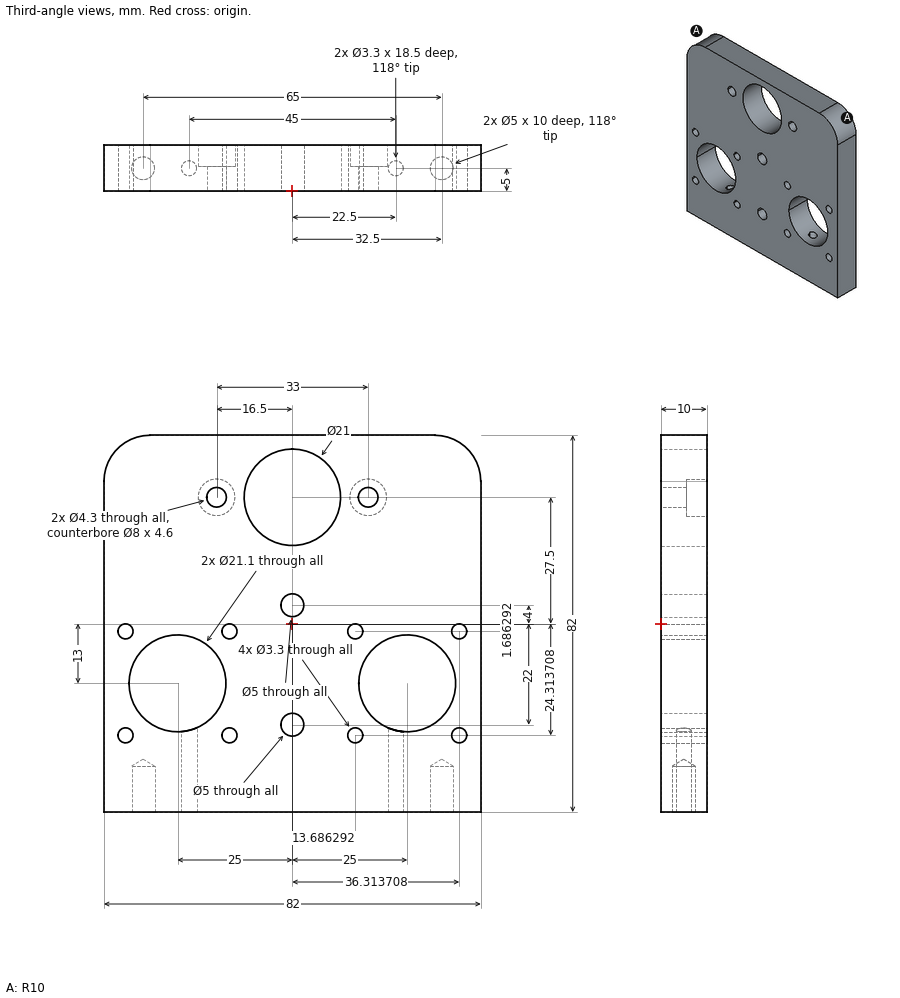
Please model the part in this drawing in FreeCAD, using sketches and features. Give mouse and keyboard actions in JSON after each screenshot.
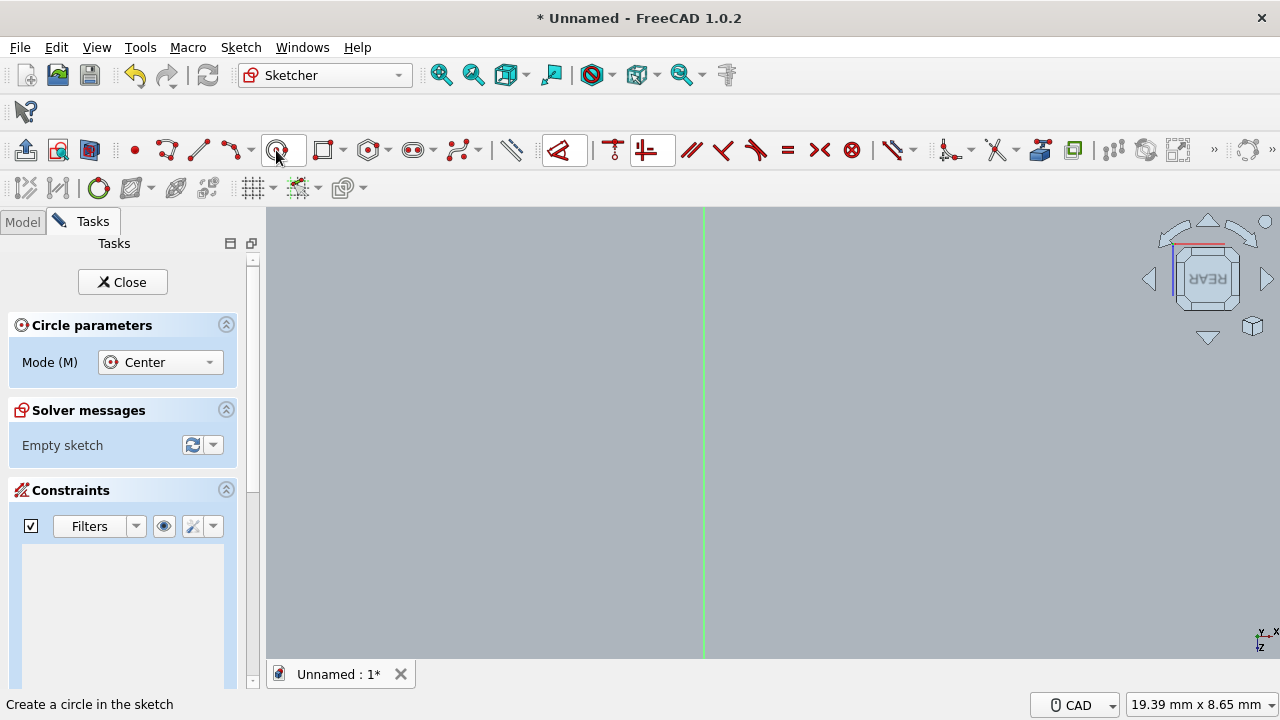
{"action": "left_click", "coordinate": [704, 426]}
{"action": "left_click", "coordinate": [797, 333]}
{"action": "key", "text": "Escape"}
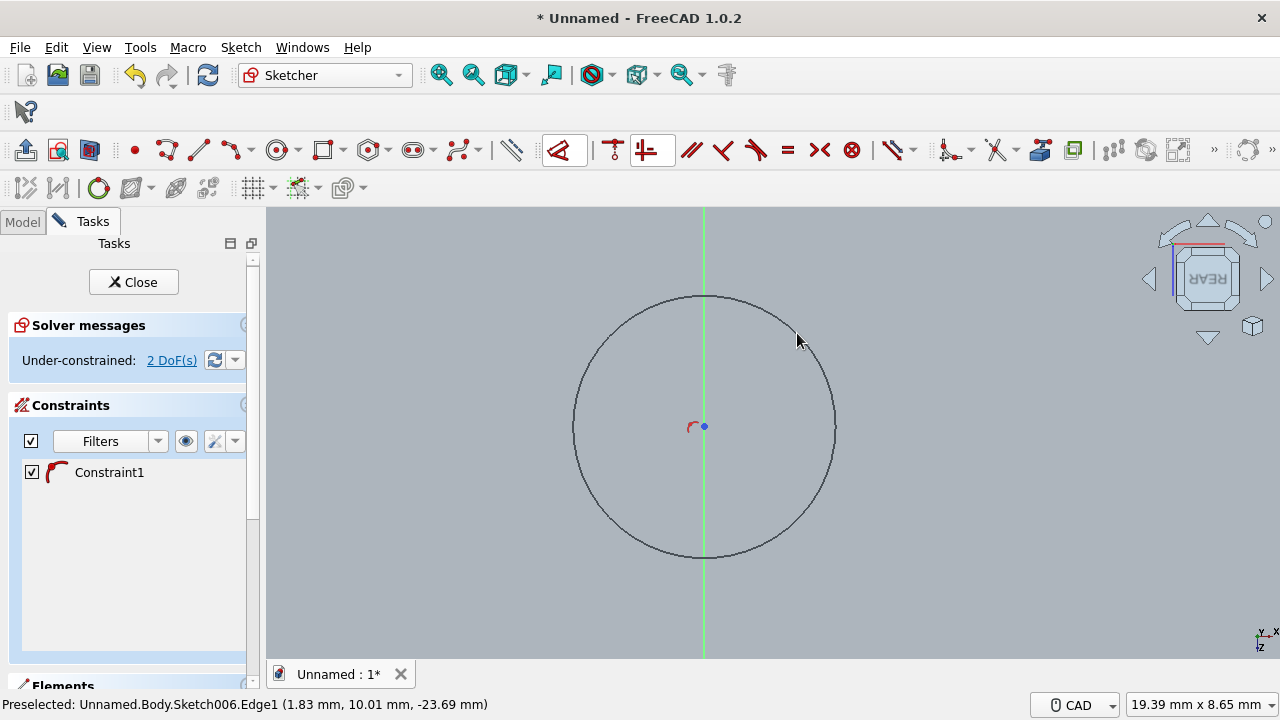
{"action": "left_click", "coordinate": [797, 334]}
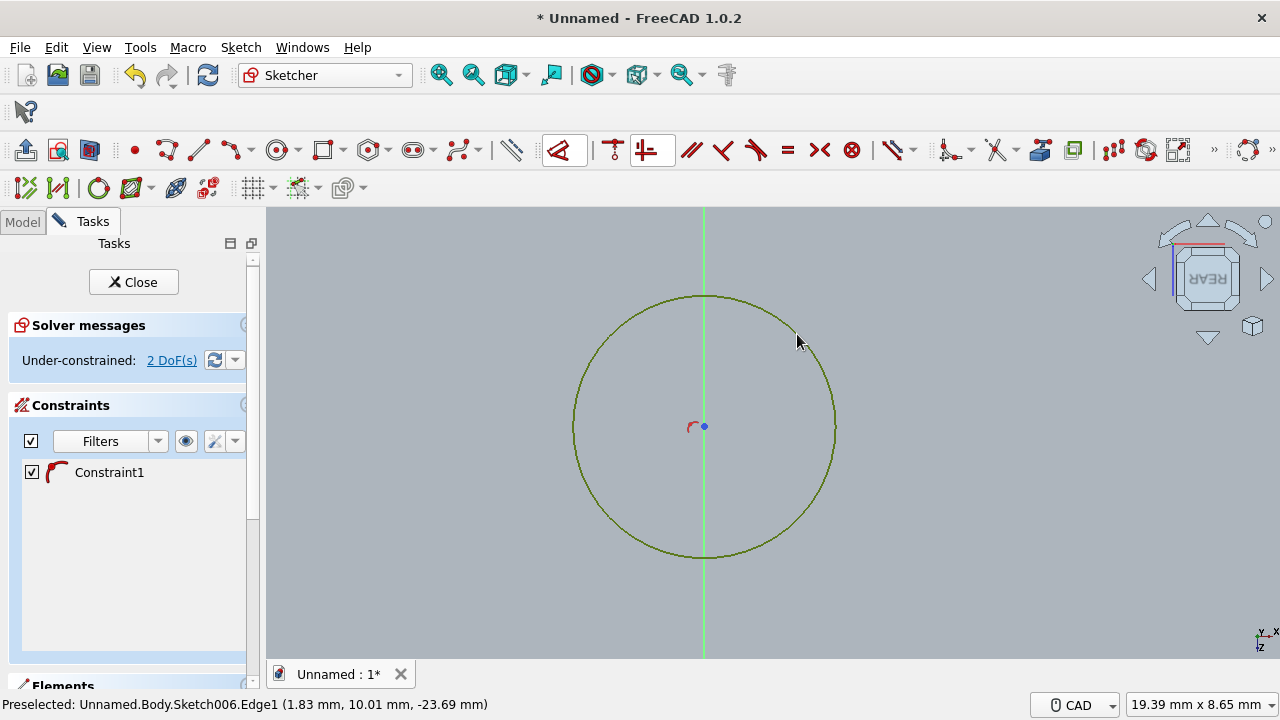
{"action": "left_click", "coordinate": [582, 150]}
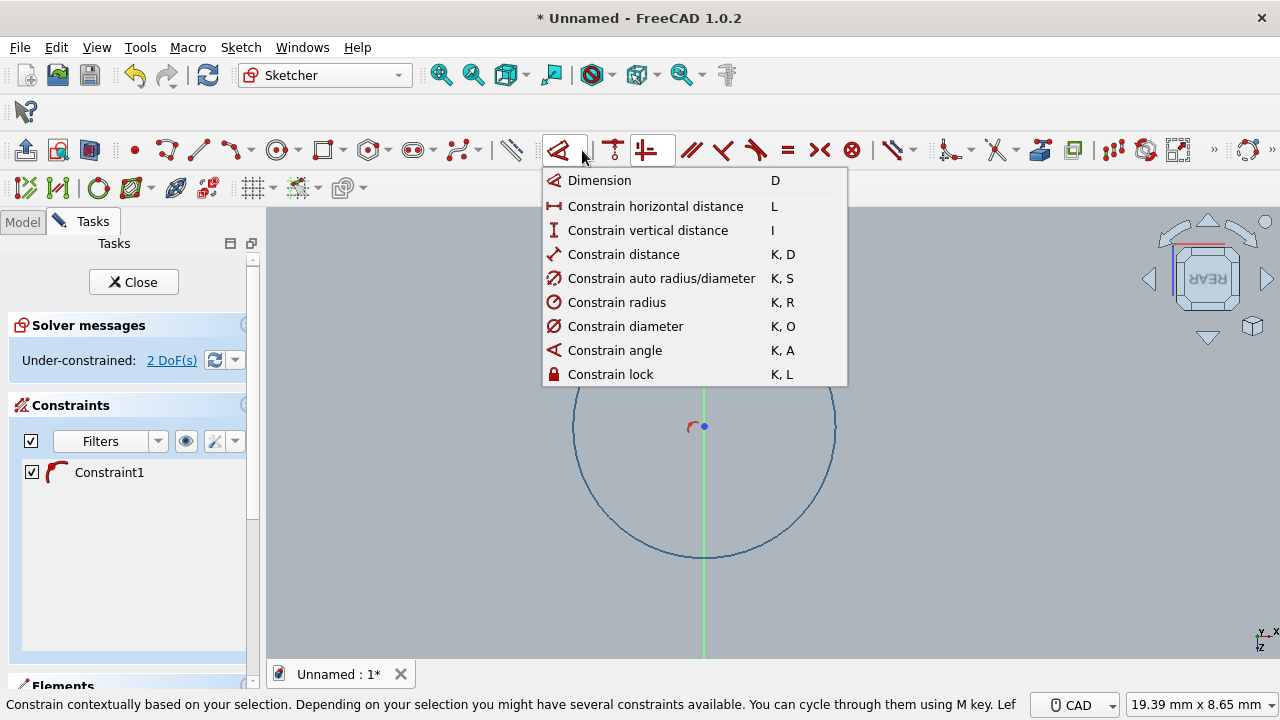
{"action": "left_click", "coordinate": [695, 326]}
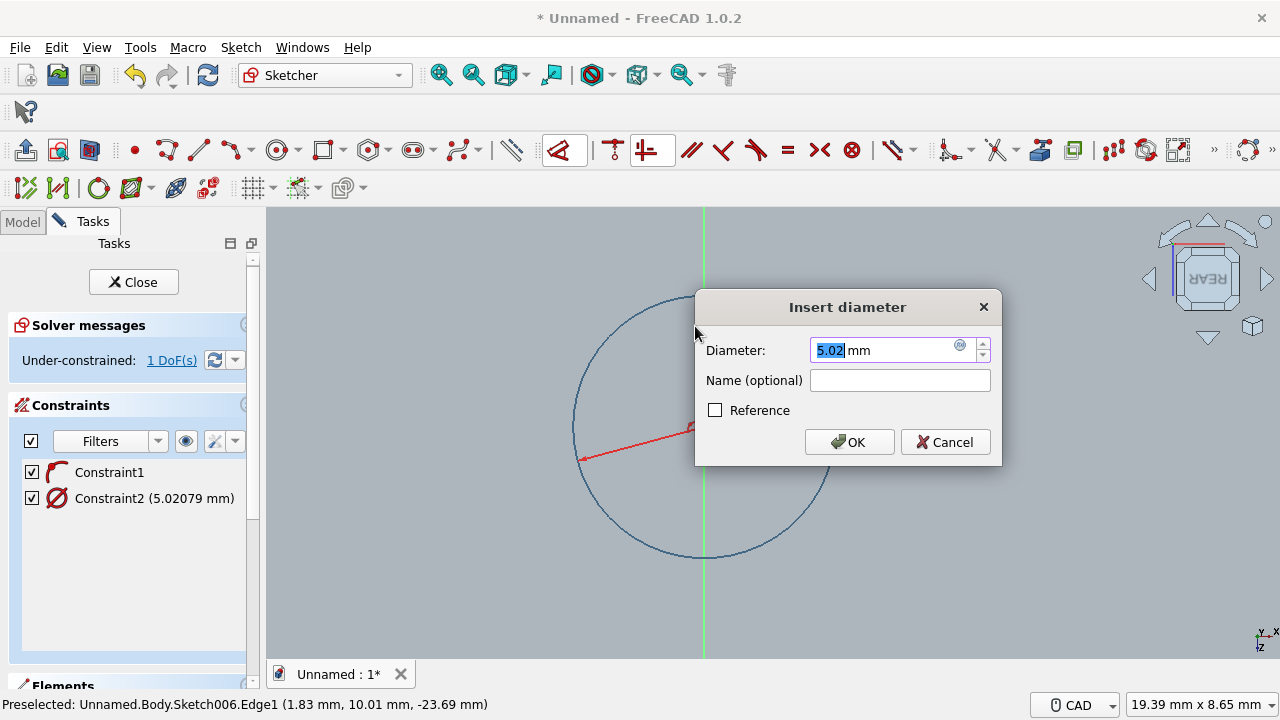
{"action": "type", "text": "5"}
{"action": "key", "text": "Return"}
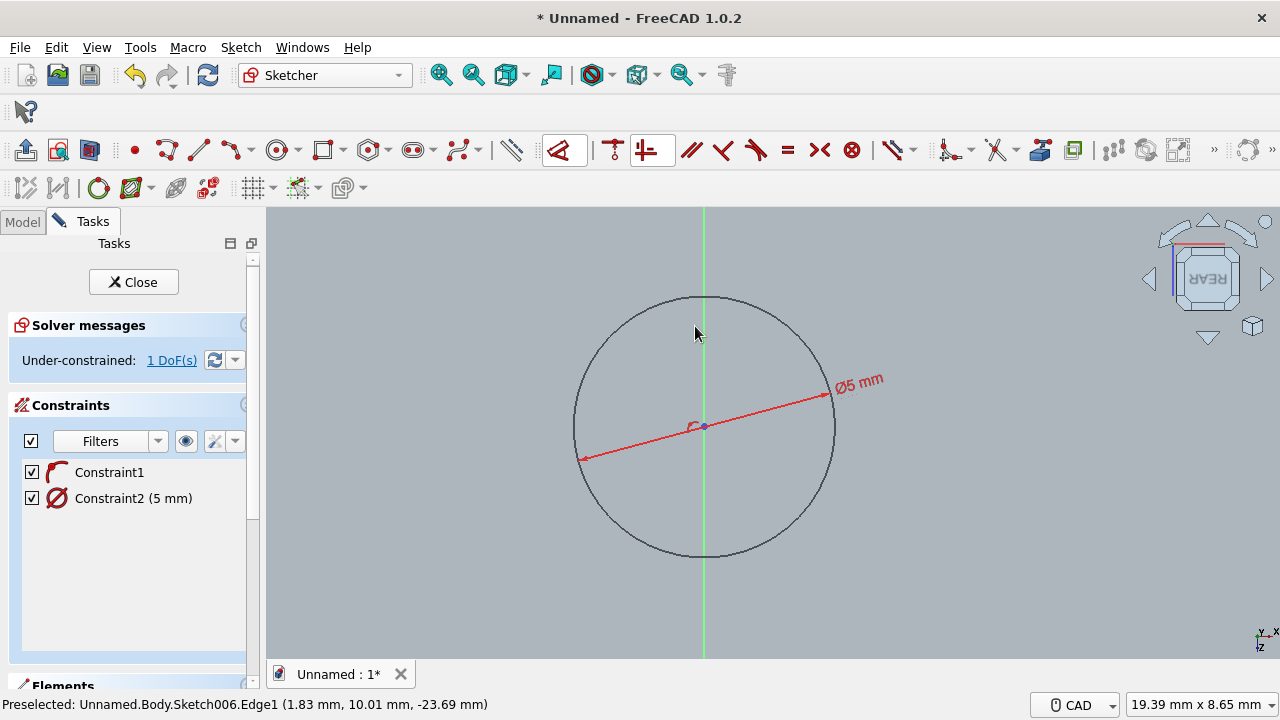
{"action": "left_click", "coordinate": [704, 427]}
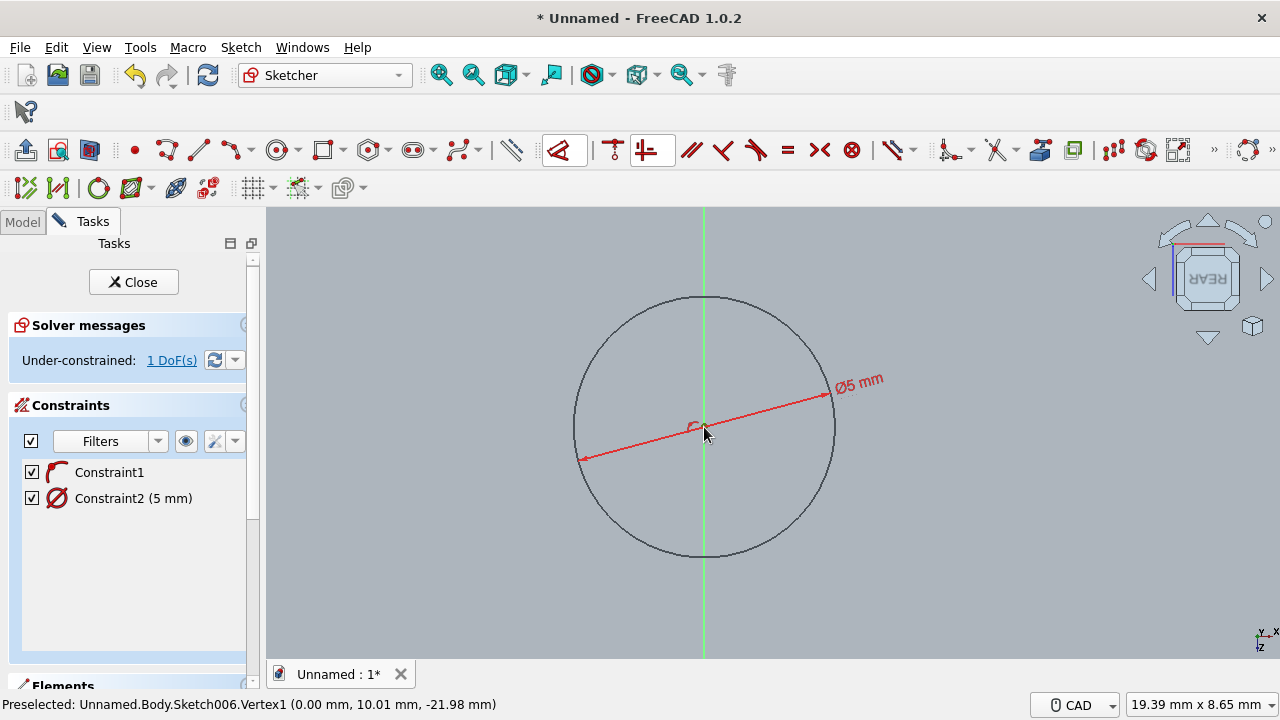
{"action": "left_click", "coordinate": [582, 150]}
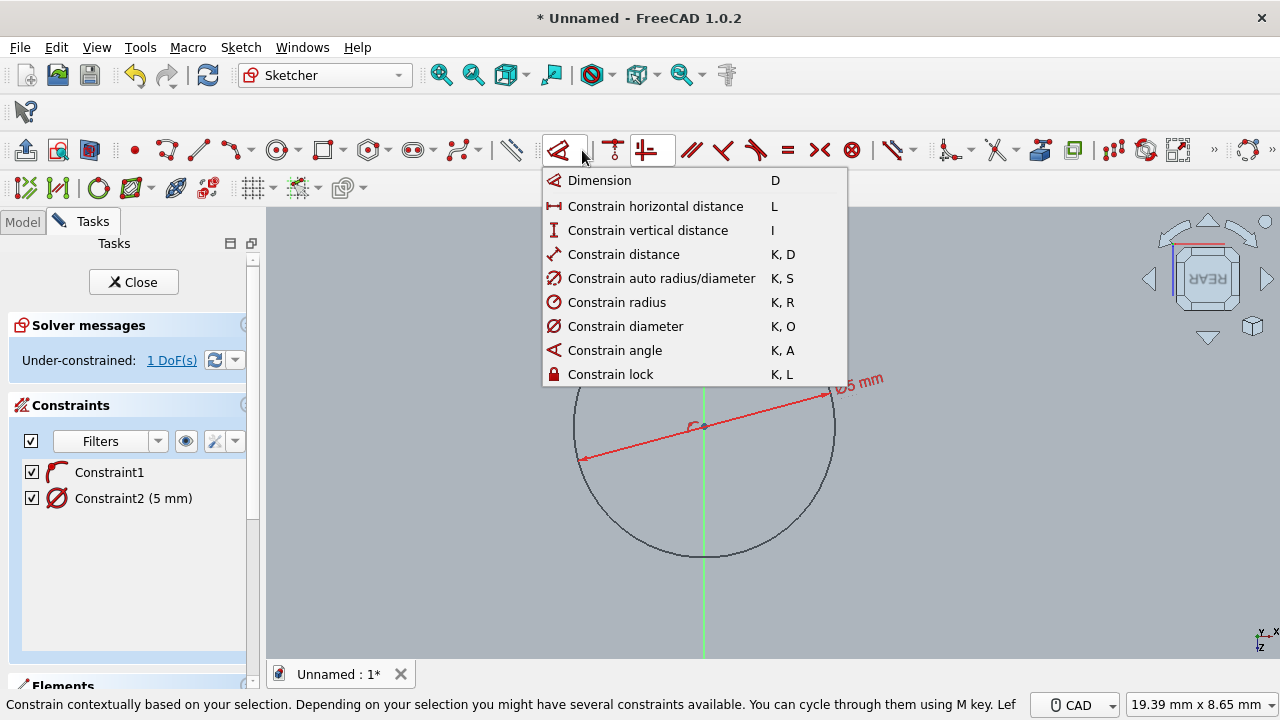
{"action": "left_click", "coordinate": [695, 230]}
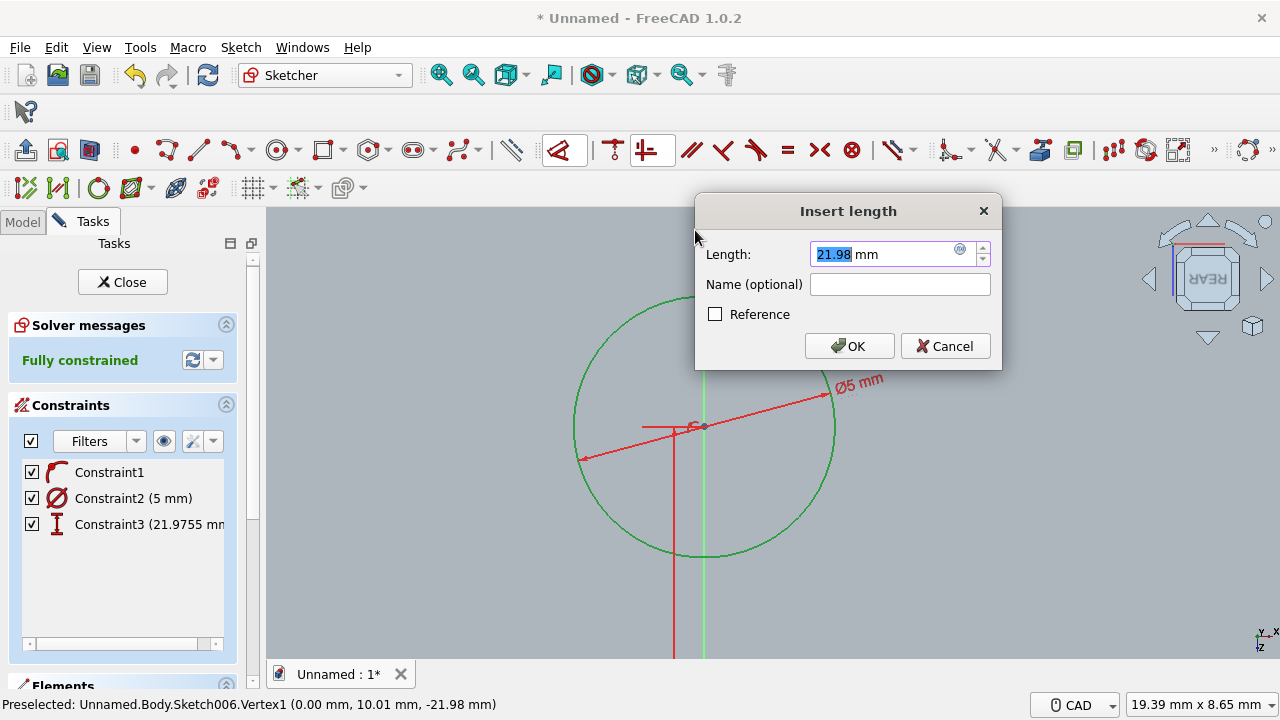
{"action": "type", "text": "22"}
{"action": "key", "text": "Return"}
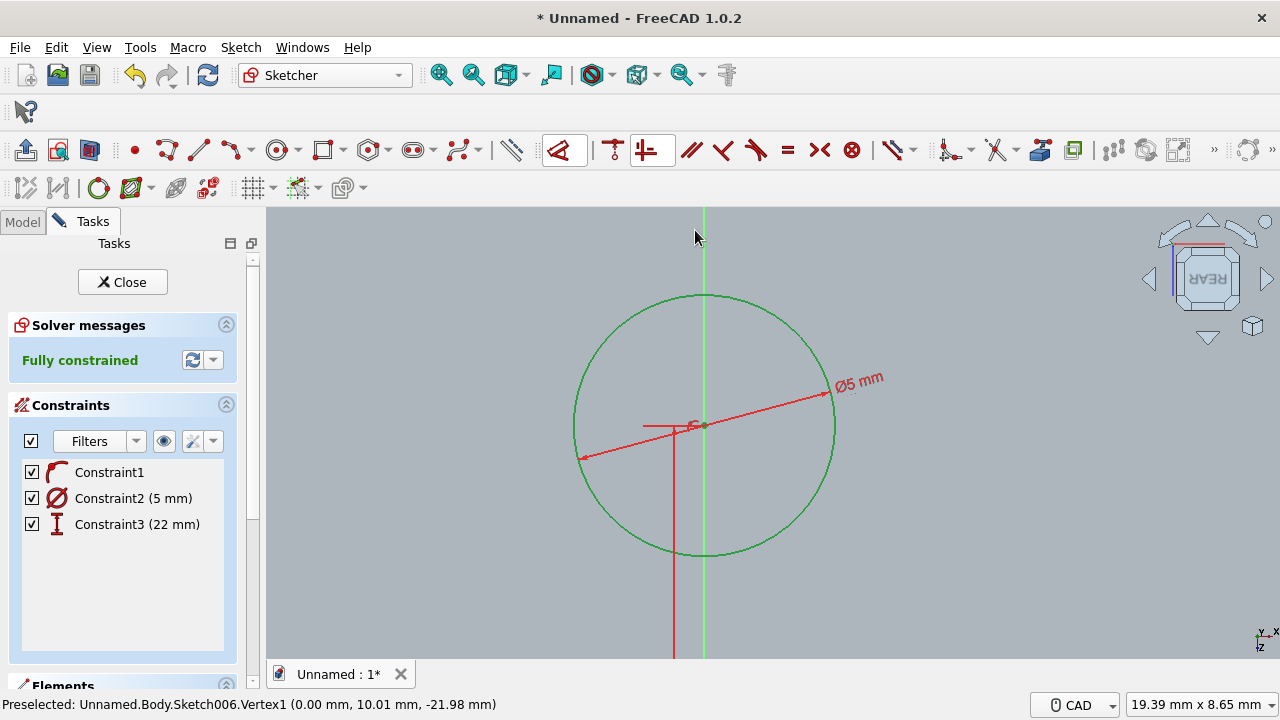
{"action": "left_click", "coordinate": [123, 282]}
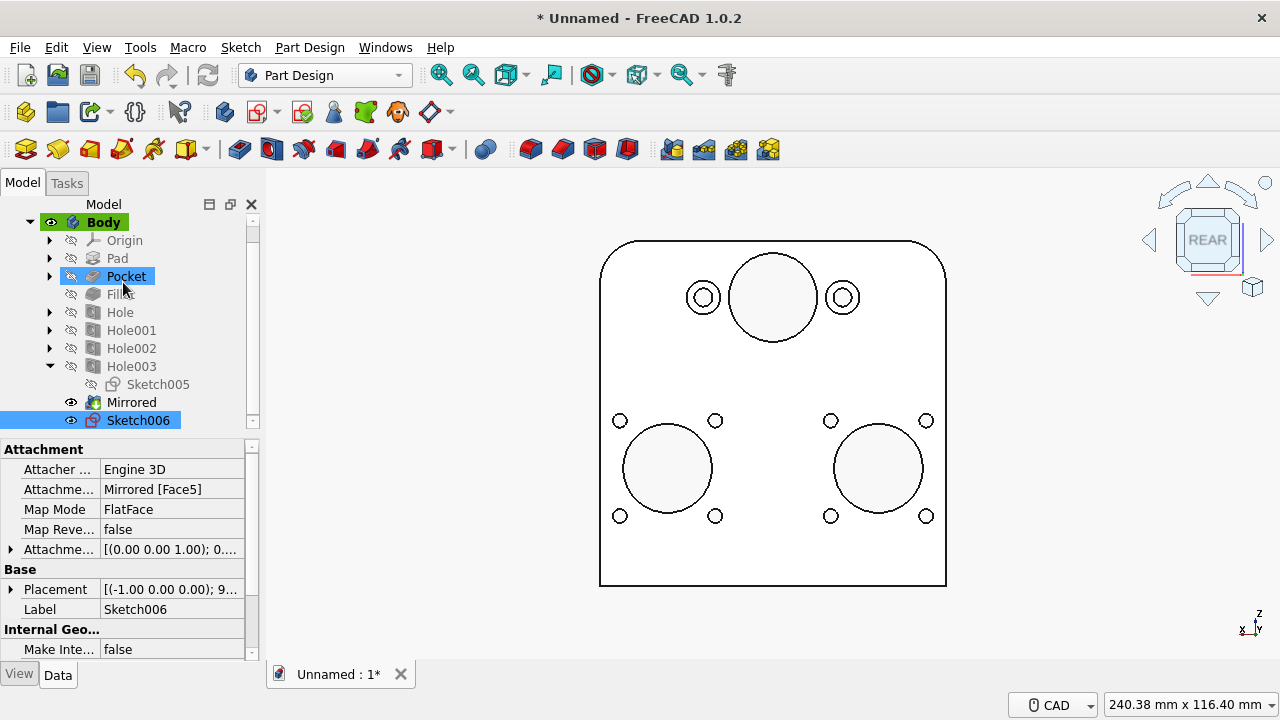
{"action": "left_click", "coordinate": [272, 150]}